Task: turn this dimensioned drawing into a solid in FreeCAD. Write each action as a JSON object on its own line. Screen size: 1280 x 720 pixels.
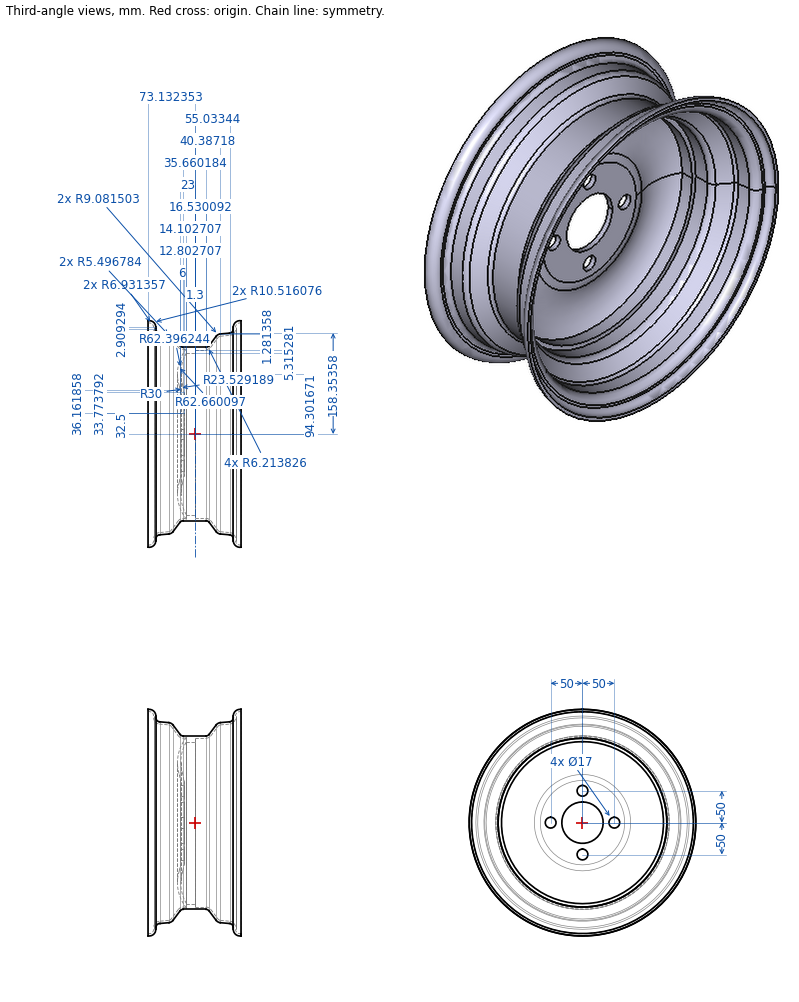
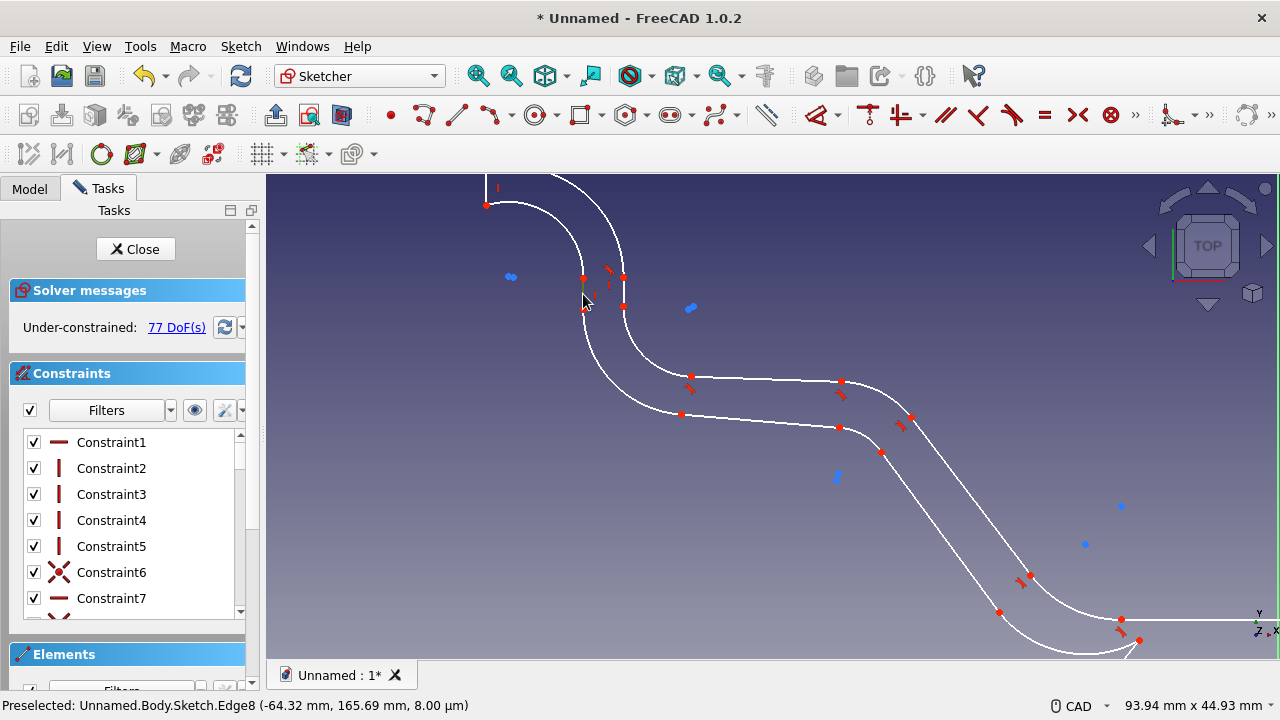
{"action": "left_click", "coordinate": [573, 238]}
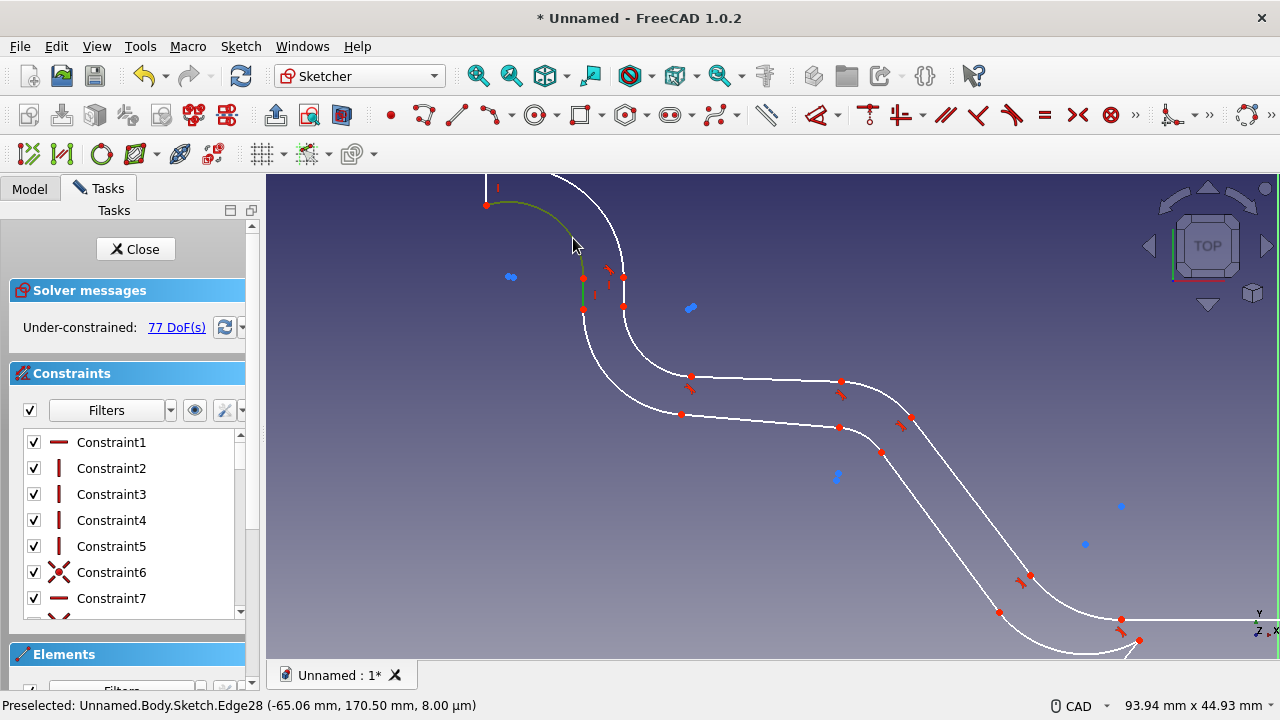
{"action": "key", "text": "t"}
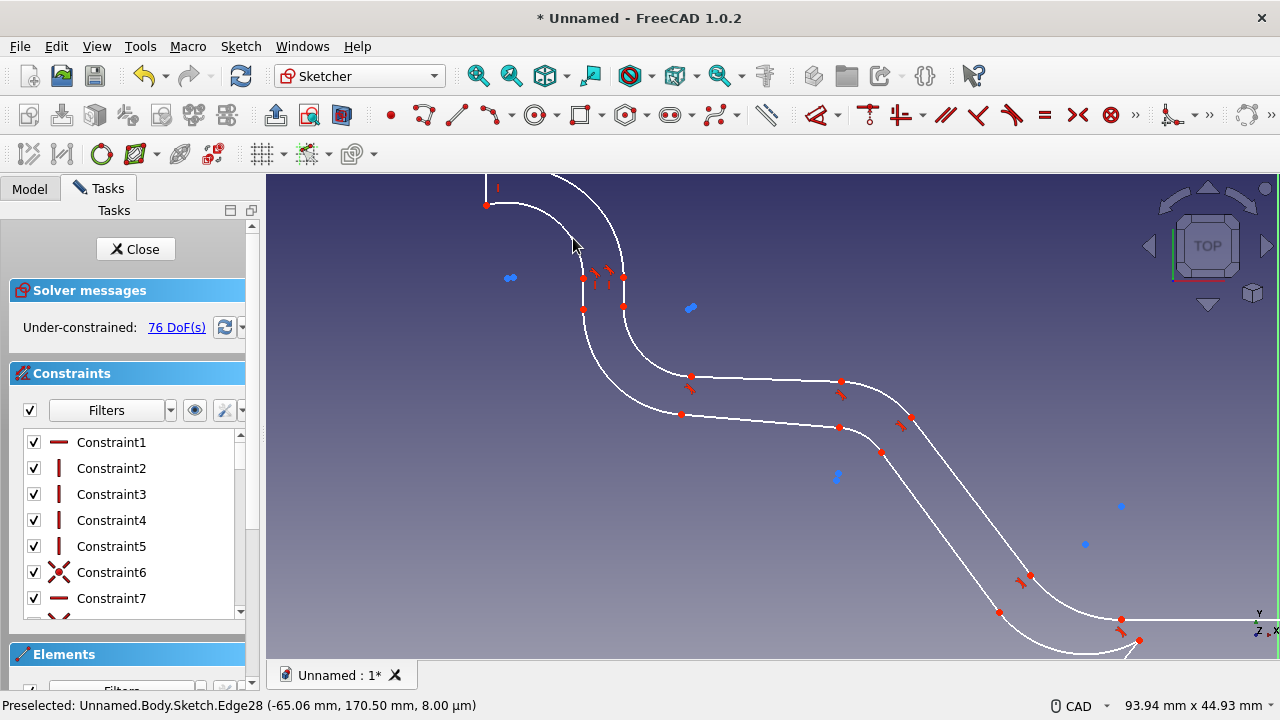
{"action": "scroll", "coordinate": [583, 288], "scroll_direction": "up", "scroll_amount": 2}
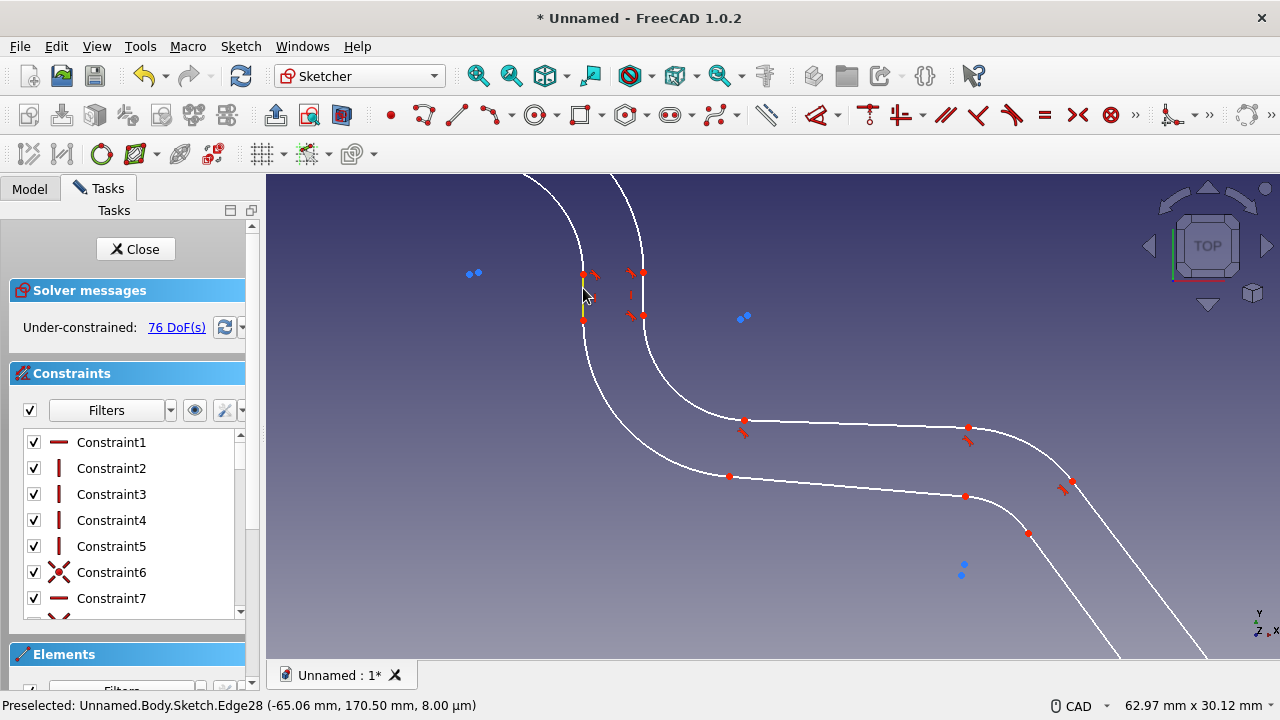
{"action": "left_click", "coordinate": [583, 288]}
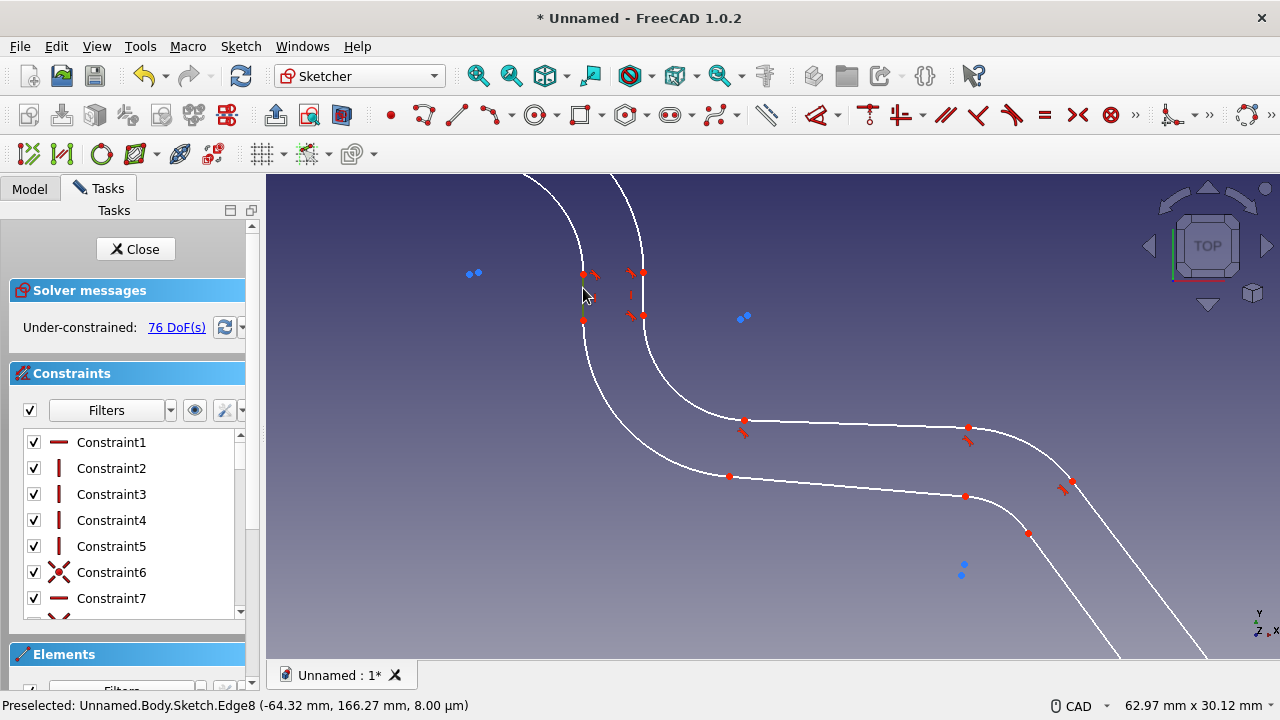
{"action": "scroll", "coordinate": [591, 277], "scroll_direction": "down", "scroll_amount": 11}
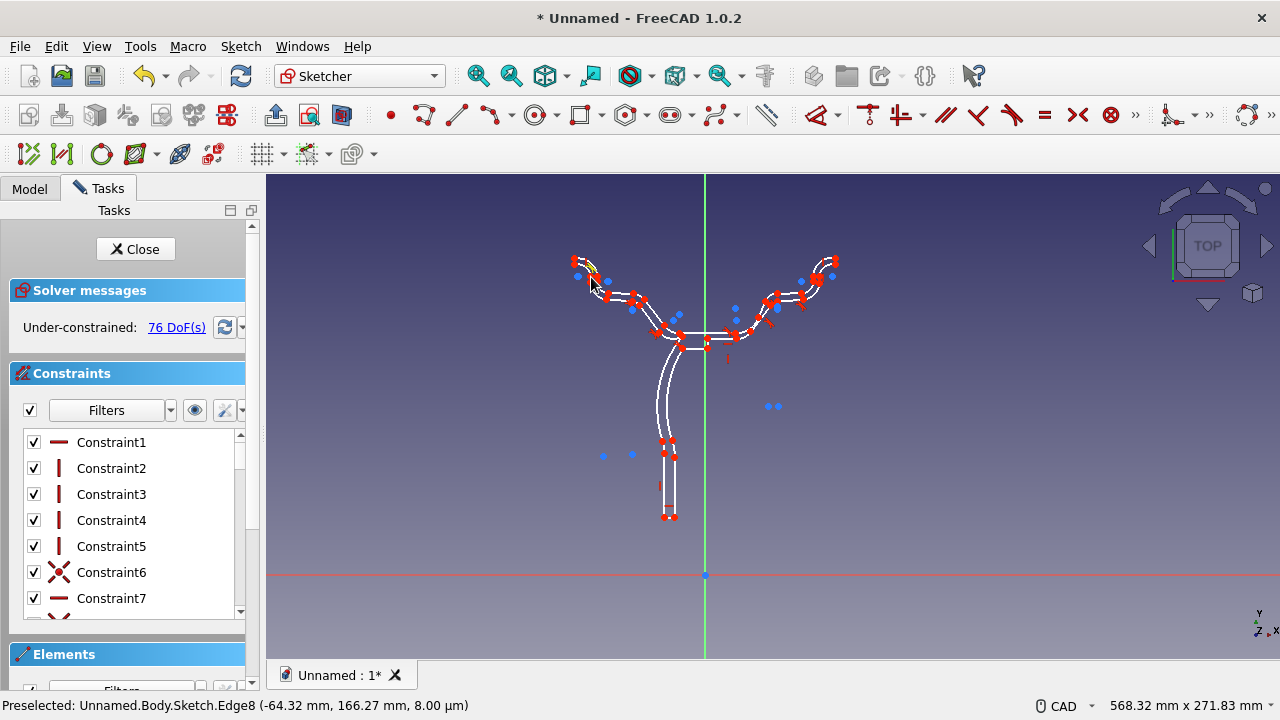
{"action": "scroll", "coordinate": [592, 290], "scroll_direction": "up", "scroll_amount": 4}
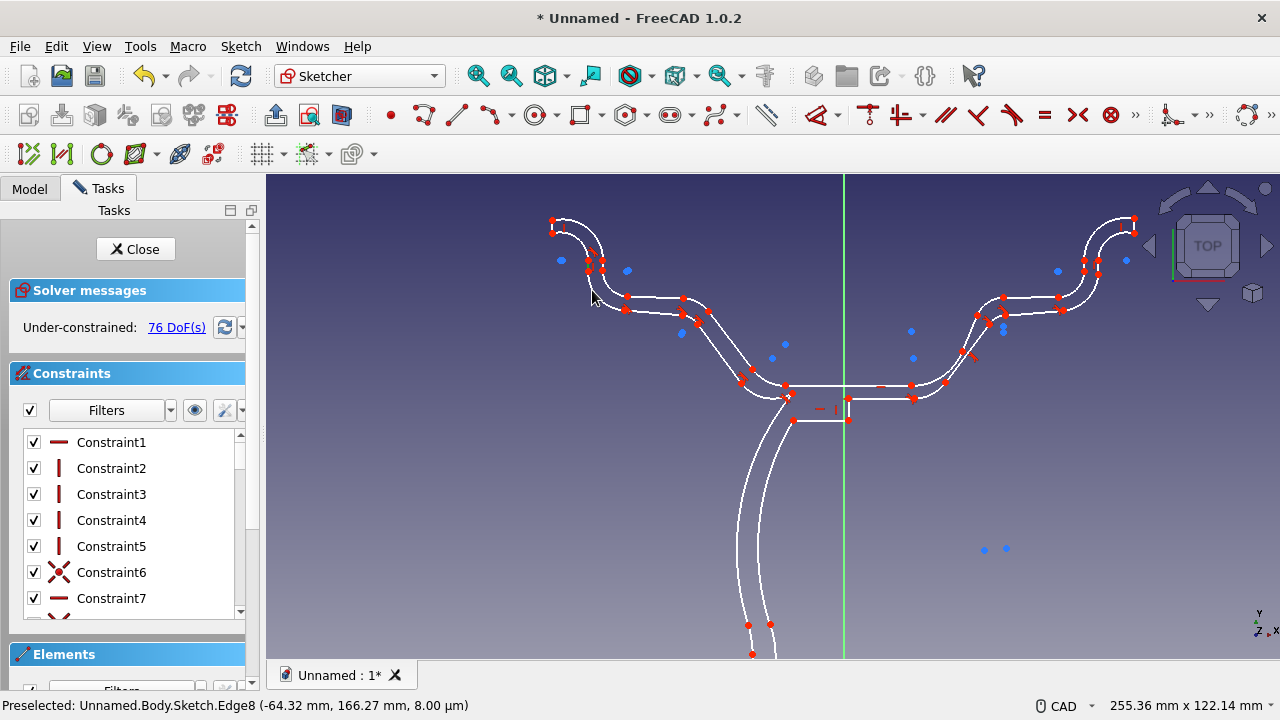
{"action": "left_click", "coordinate": [592, 289]}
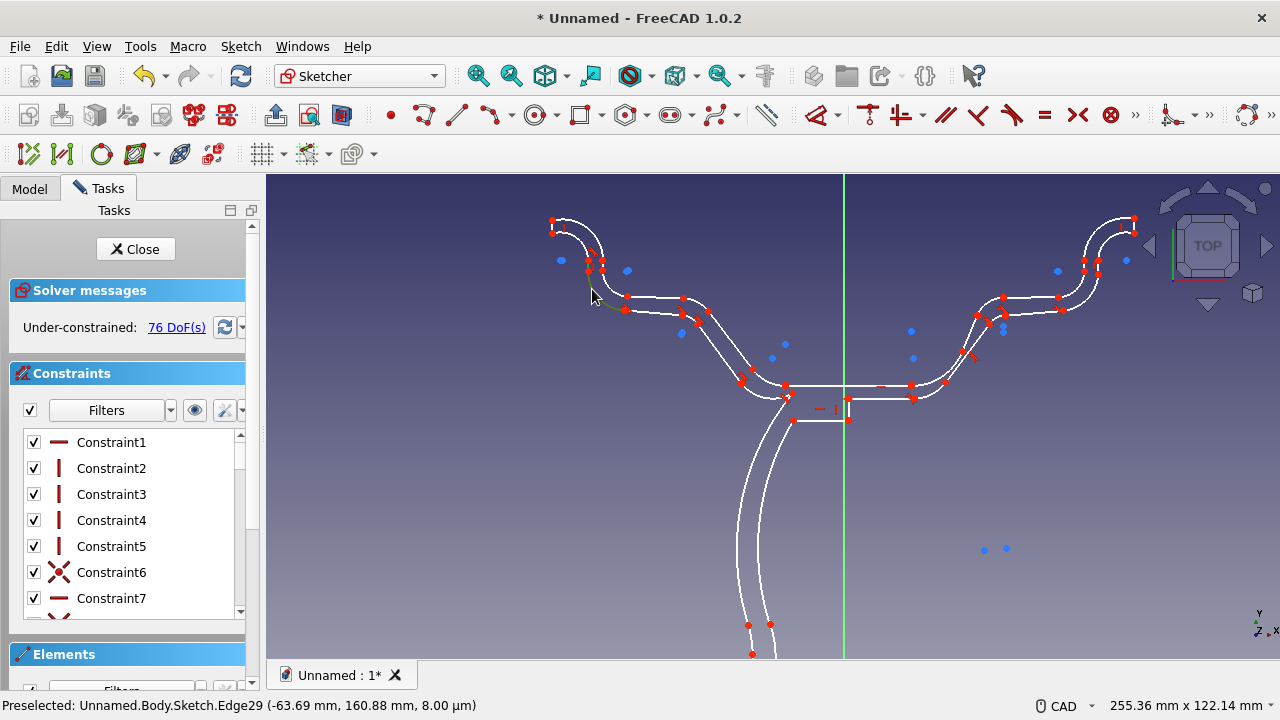
{"action": "key", "text": "t"}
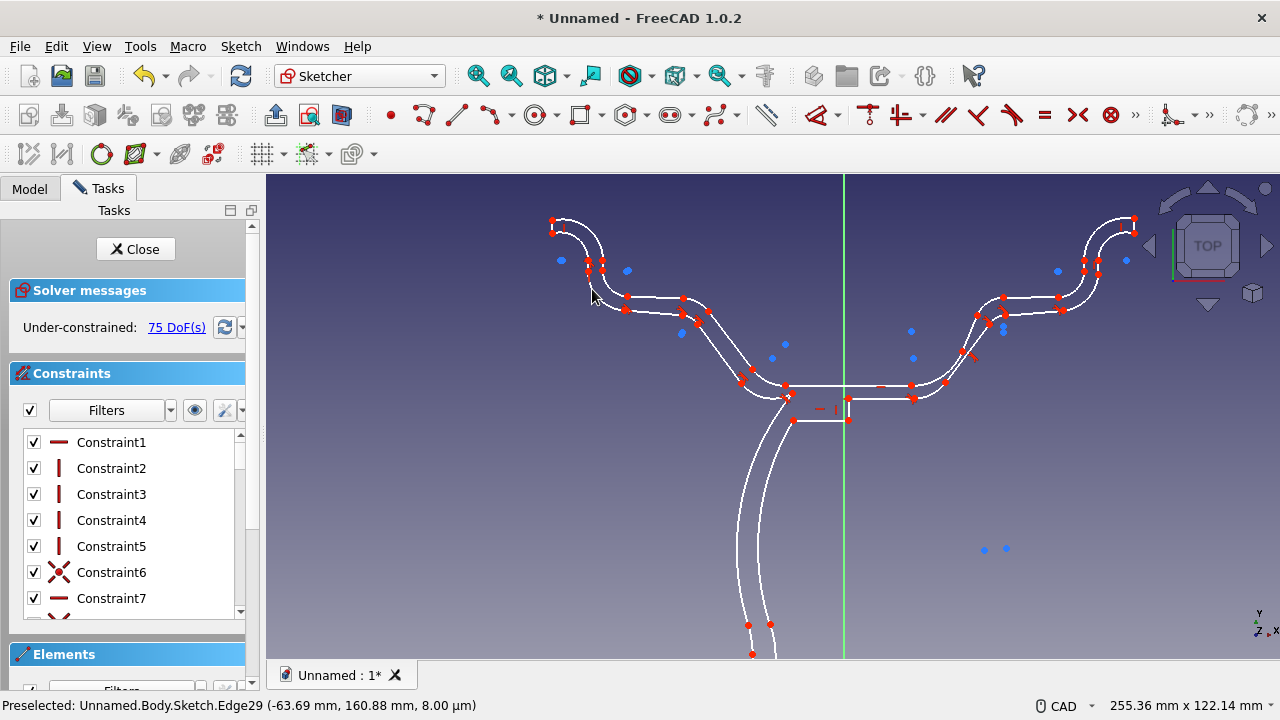
{"action": "left_click", "coordinate": [642, 312]}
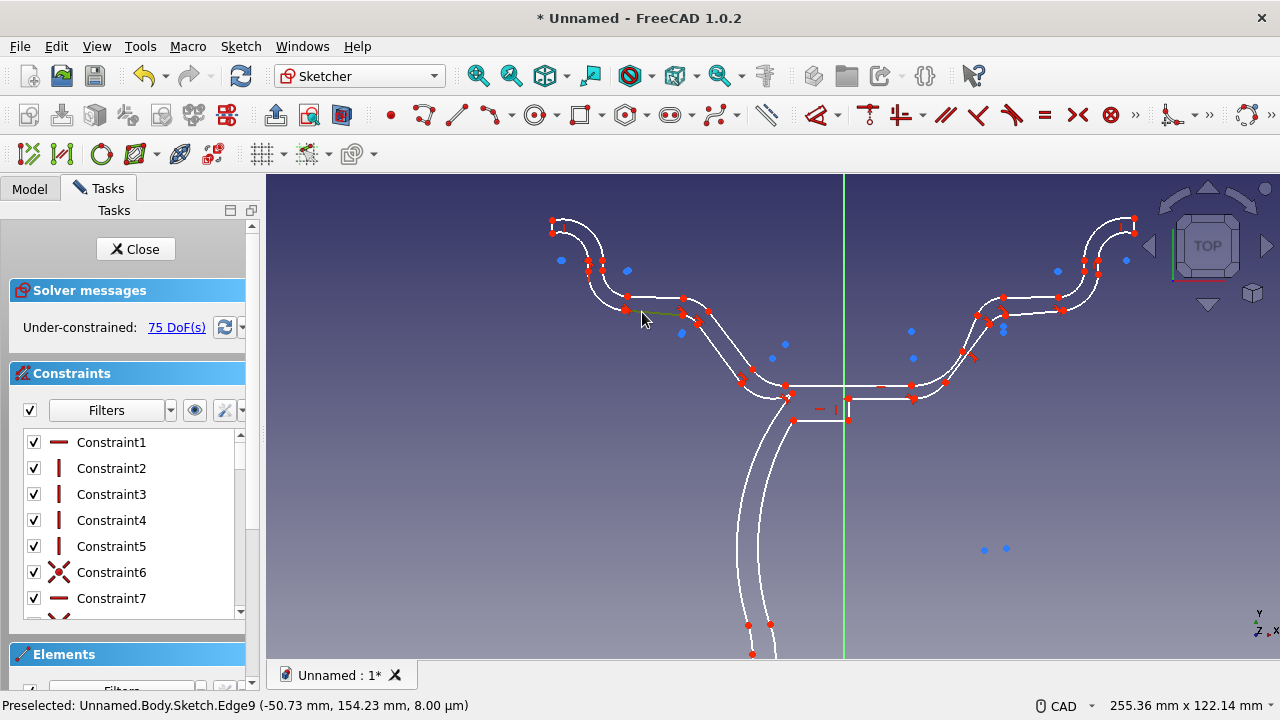
{"action": "left_click", "coordinate": [592, 289]}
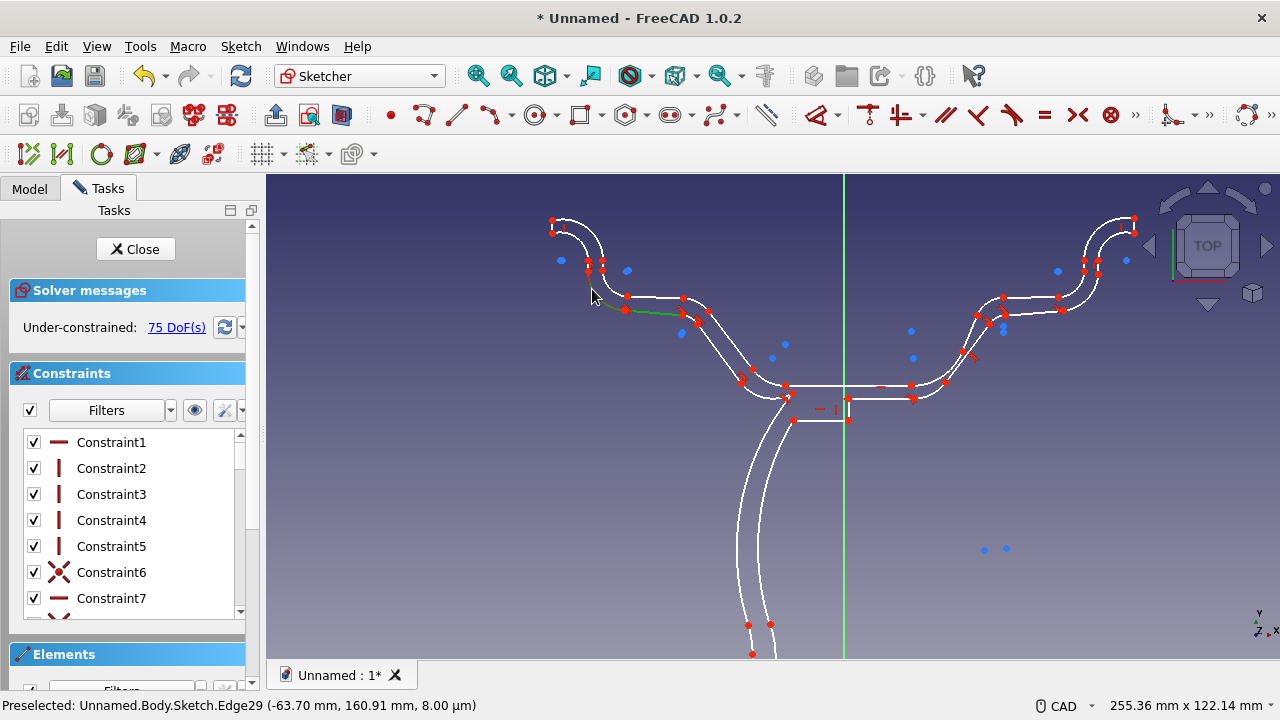
{"action": "left_click", "coordinate": [1012, 116]}